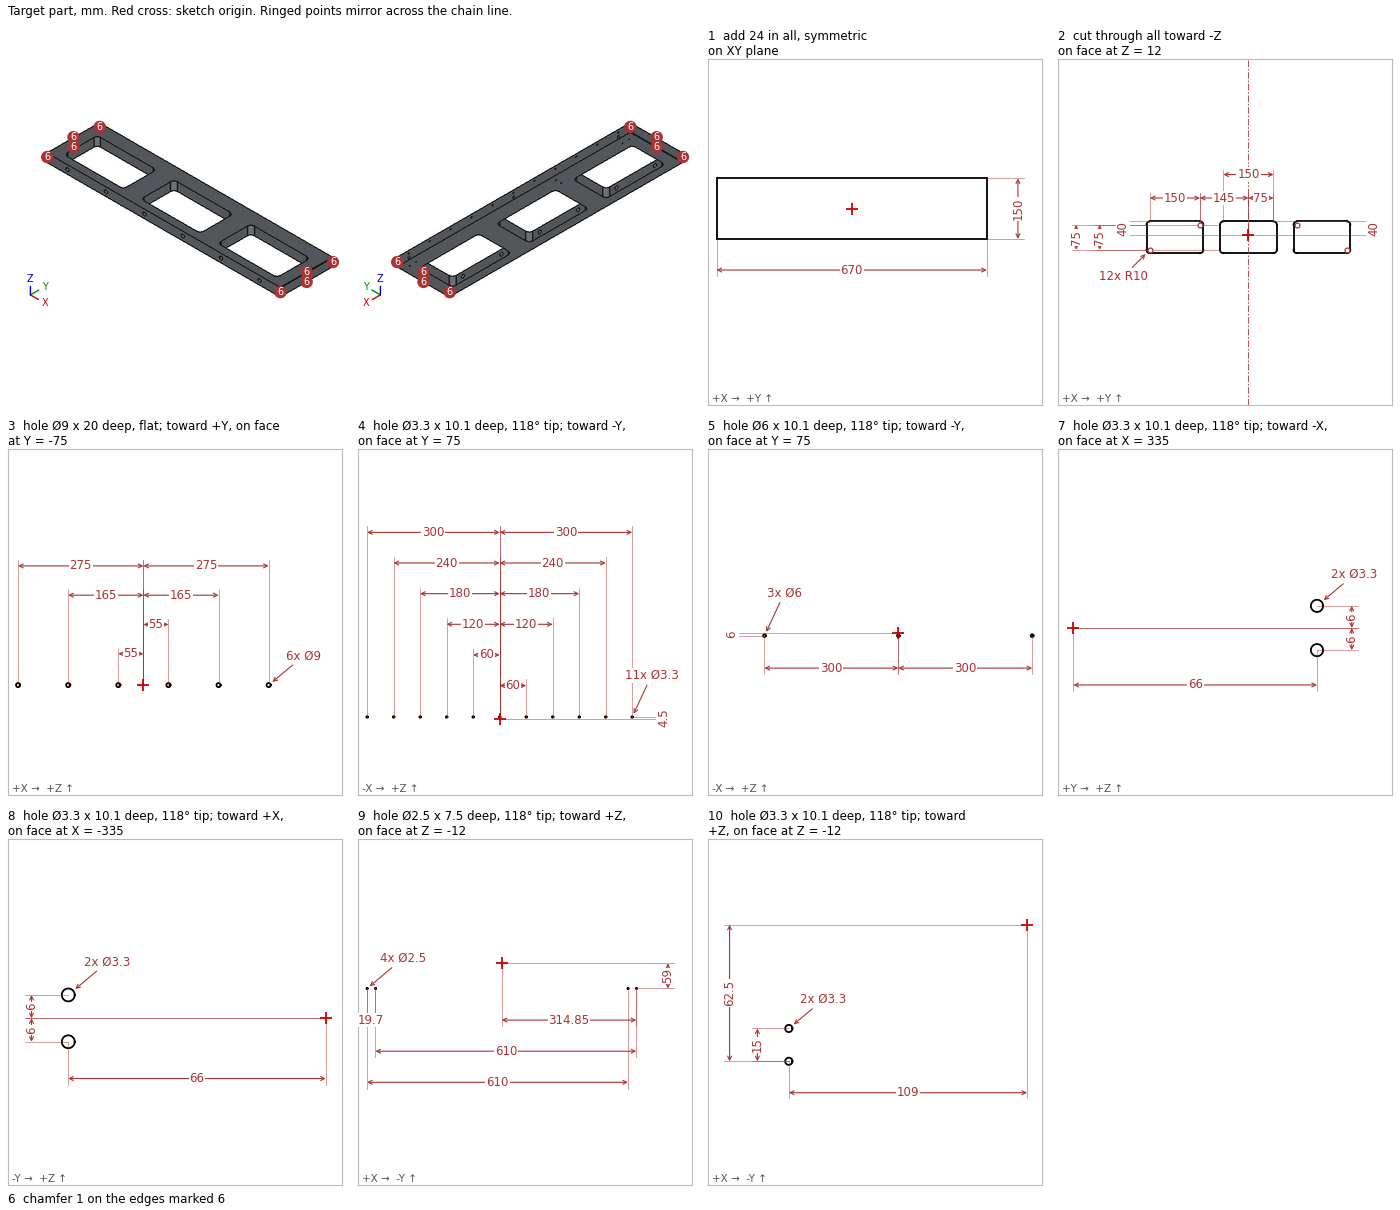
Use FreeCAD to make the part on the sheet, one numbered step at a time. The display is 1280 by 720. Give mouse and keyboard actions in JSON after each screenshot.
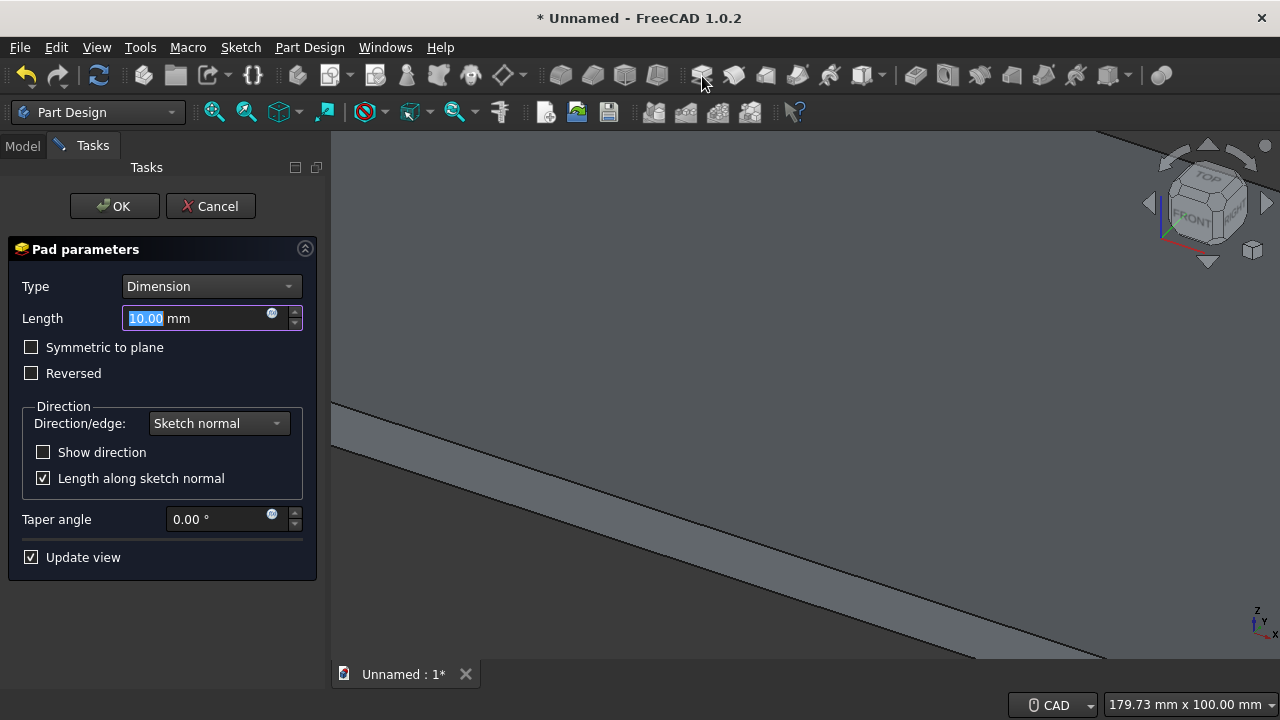
{"action": "type", "text": "24"}
{"action": "key", "text": "Tab"}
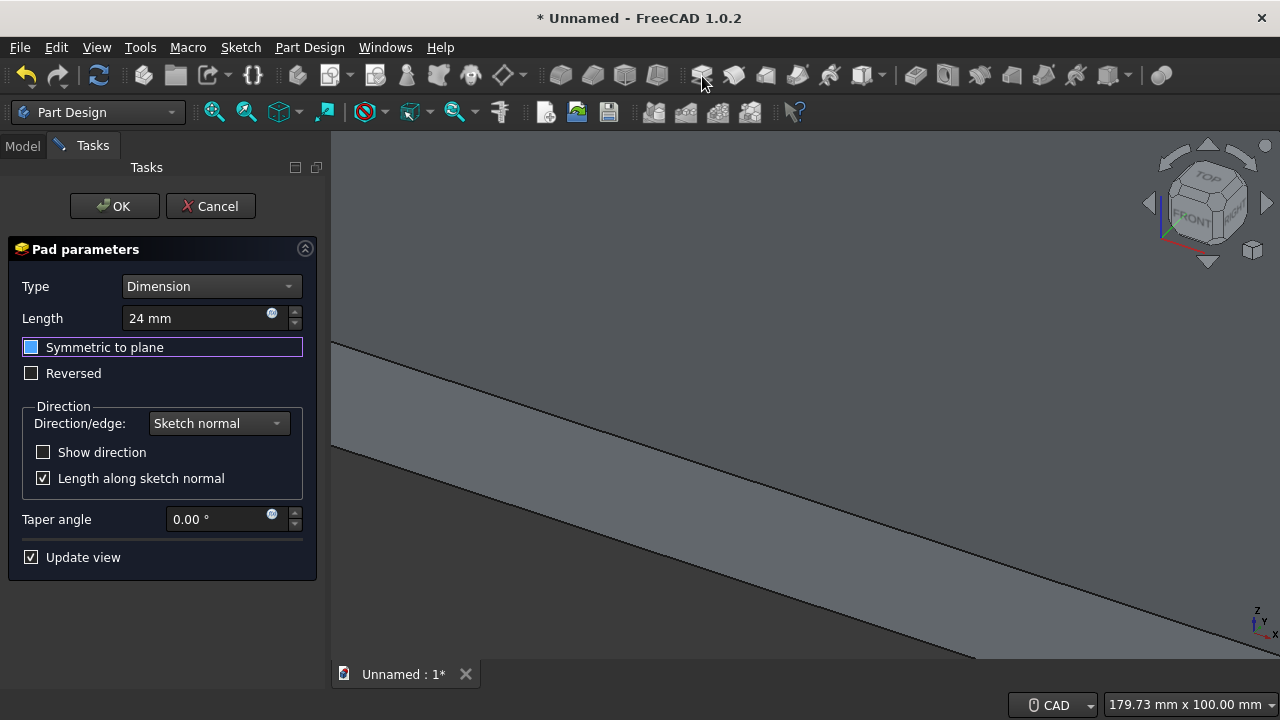
{"action": "left_click", "coordinate": [30, 347]}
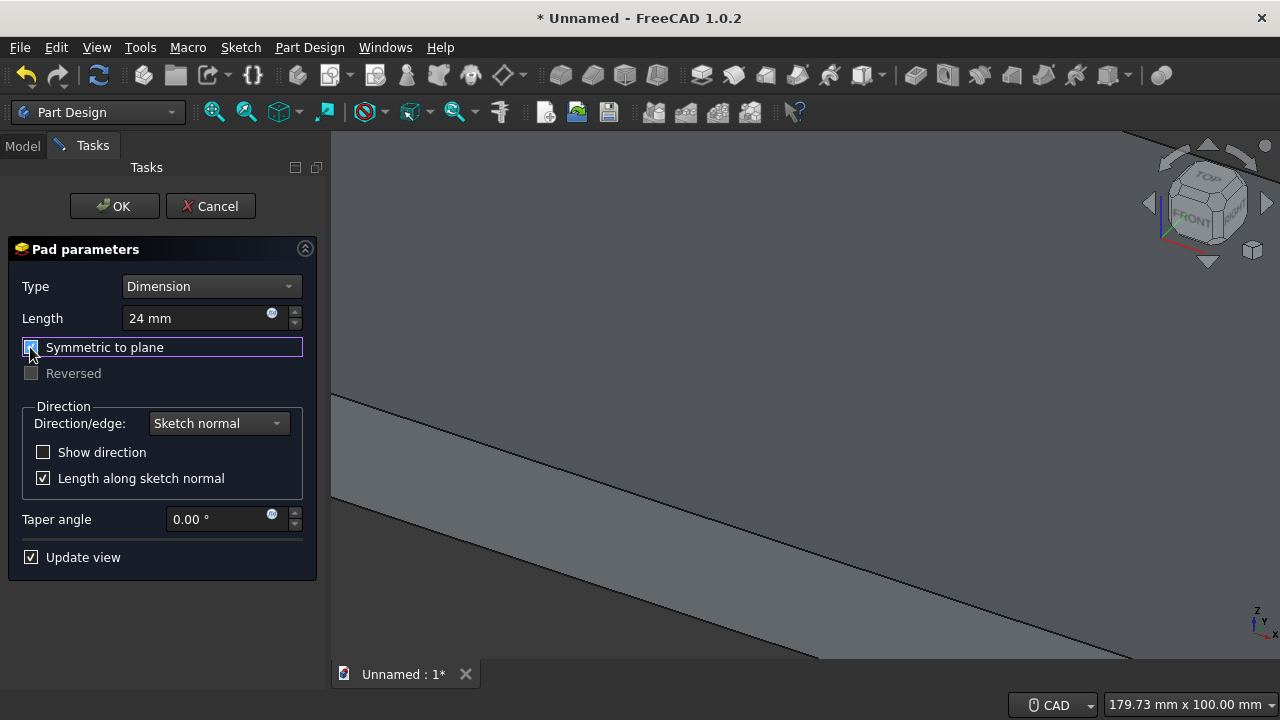
{"action": "left_click", "coordinate": [115, 206]}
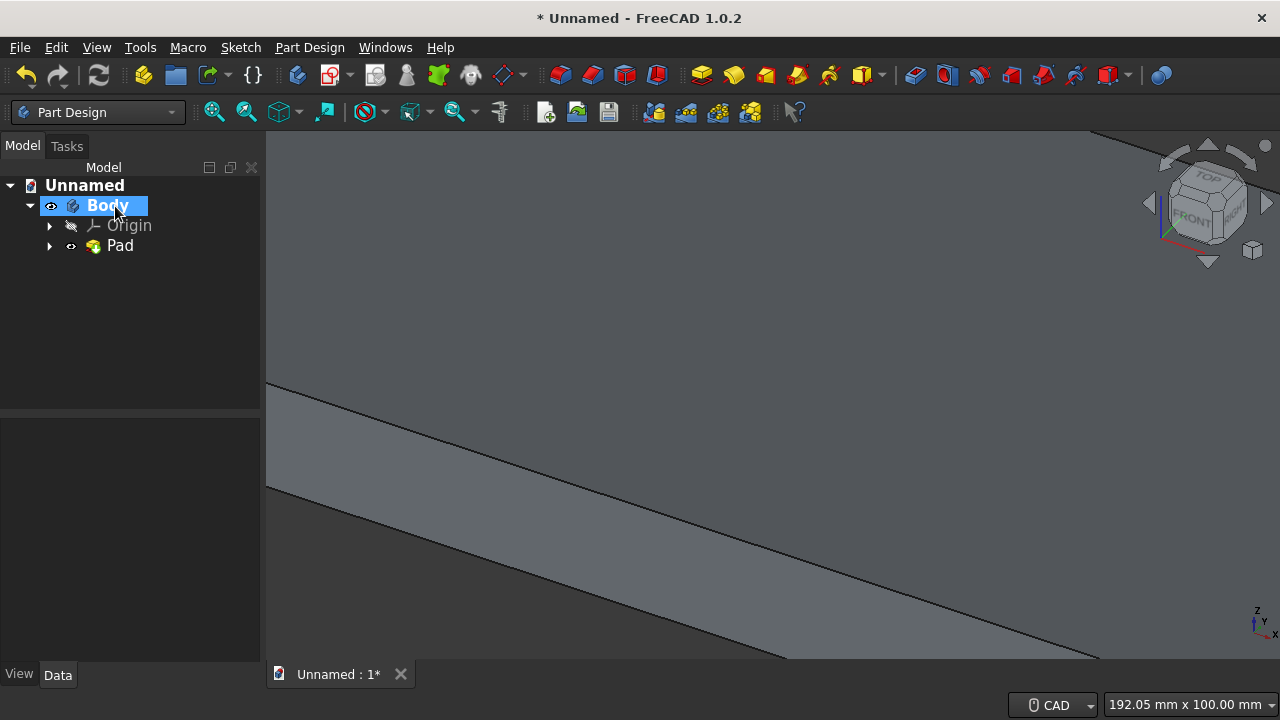
{"action": "left_click", "coordinate": [216, 112]}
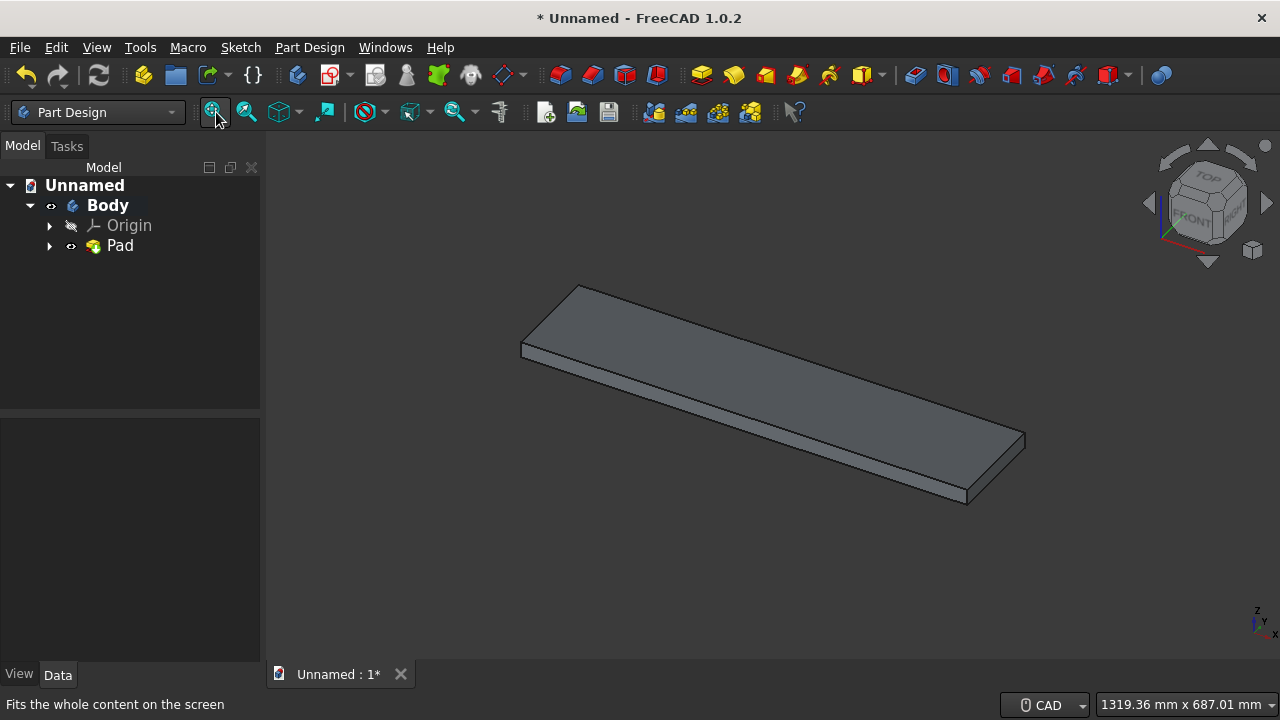
{"action": "left_click", "coordinate": [900, 429]}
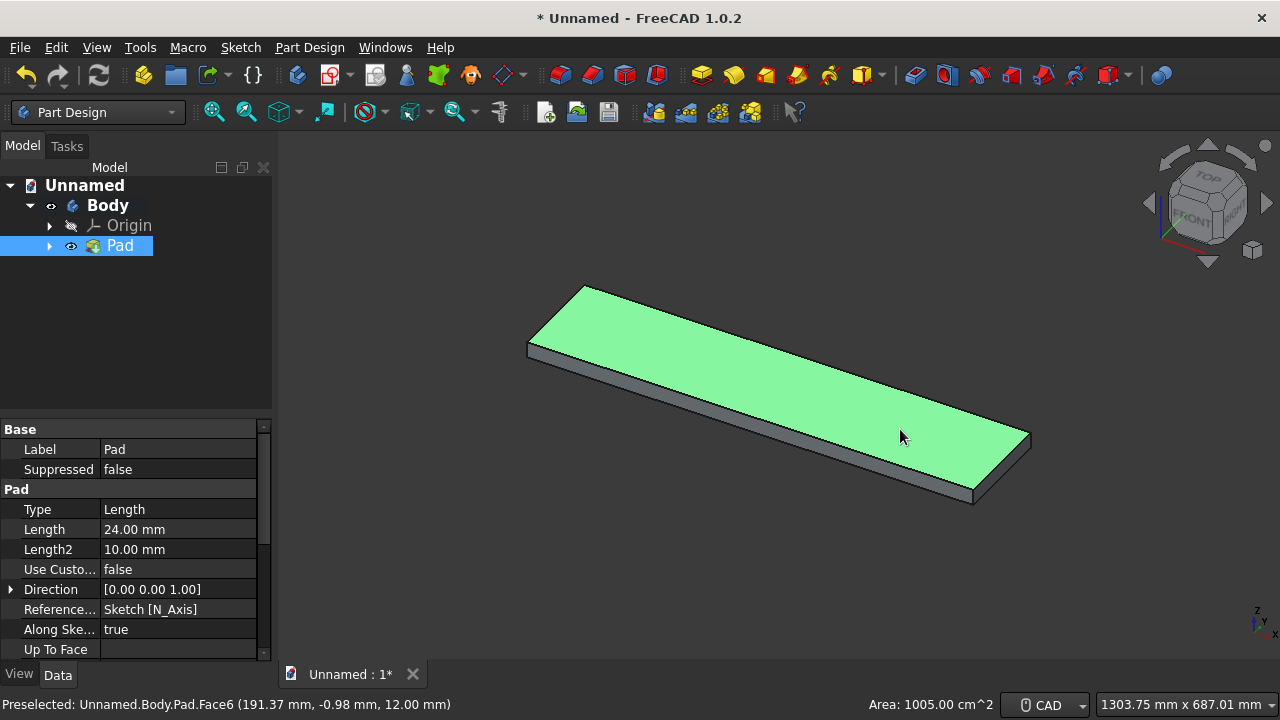
{"action": "left_click", "coordinate": [330, 76]}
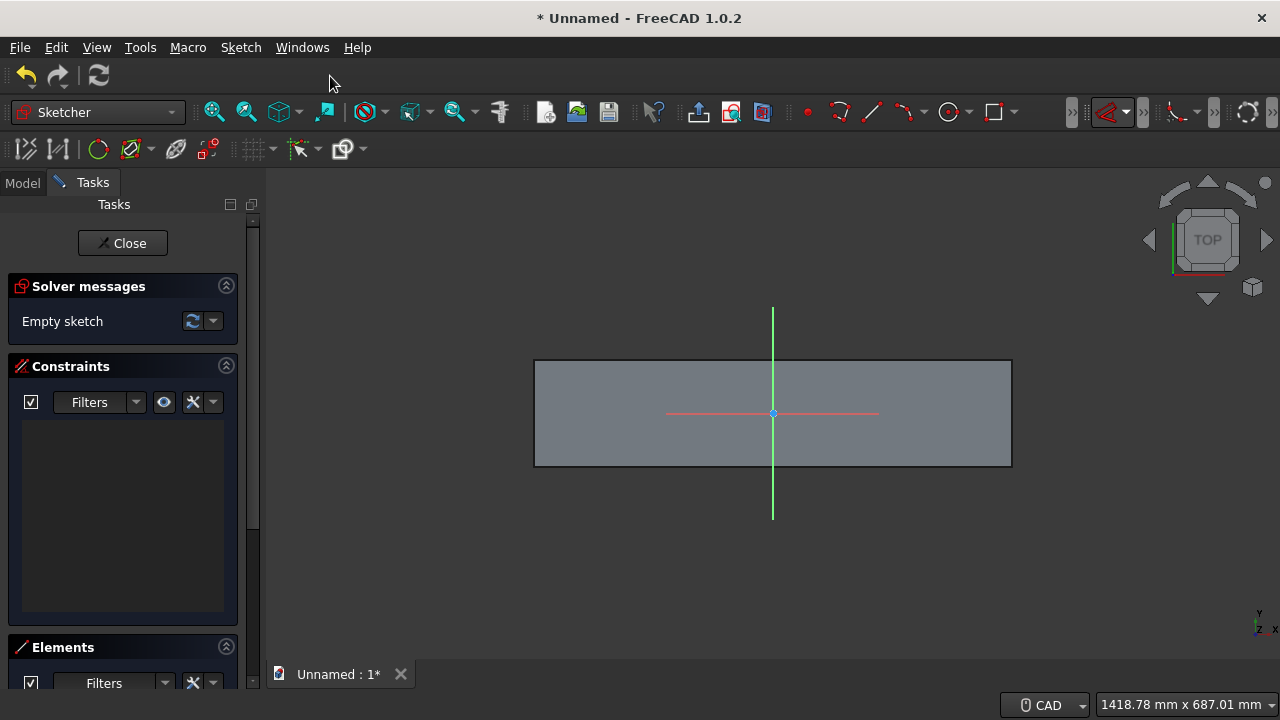
{"action": "left_click", "coordinate": [872, 112]}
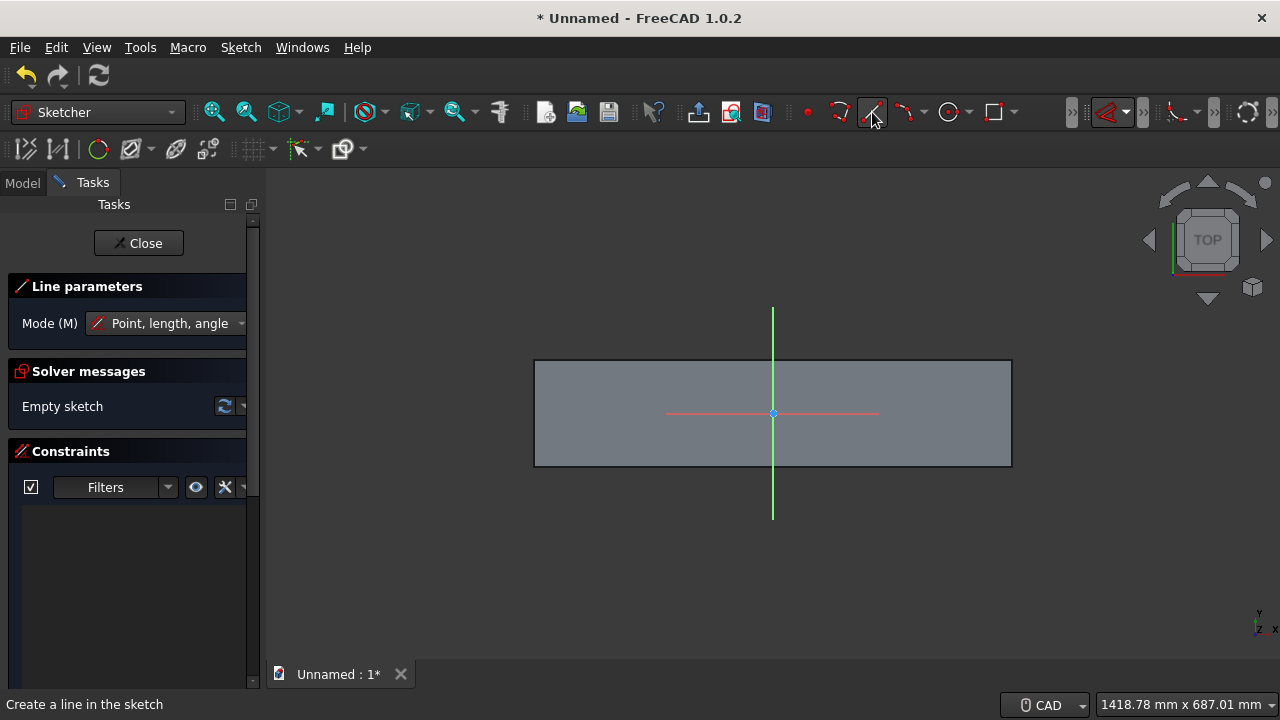
{"action": "left_click", "coordinate": [669, 385]}
{"action": "left_click", "coordinate": [562, 385]}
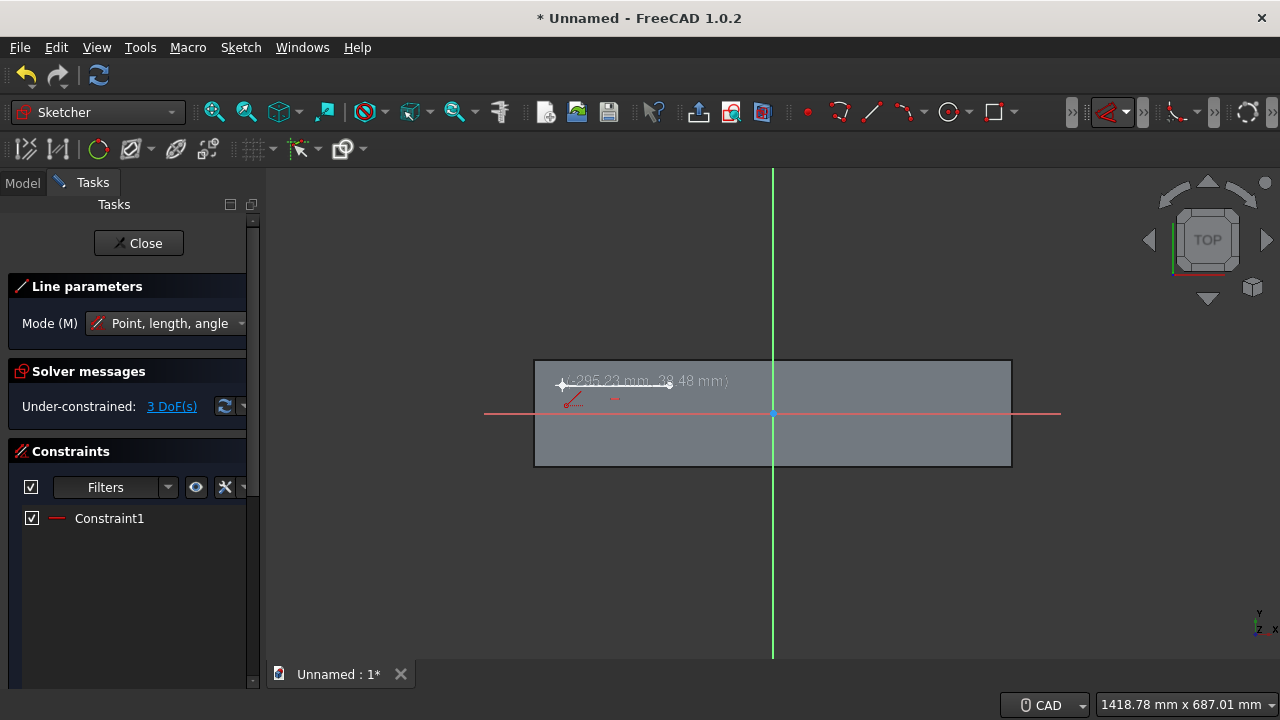
{"action": "scroll", "coordinate": [555, 392], "scroll_direction": "up", "scroll_amount": 3}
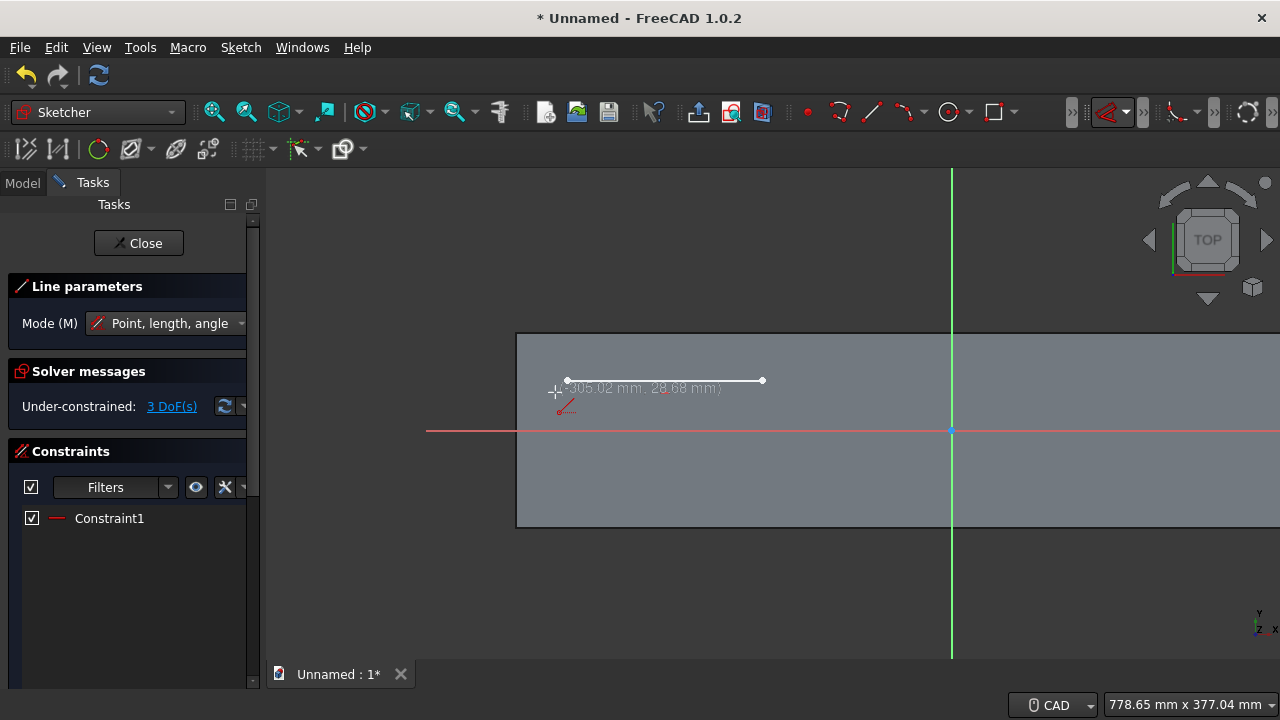
{"action": "left_click", "coordinate": [555, 392]}
{"action": "left_click", "coordinate": [555, 489]}